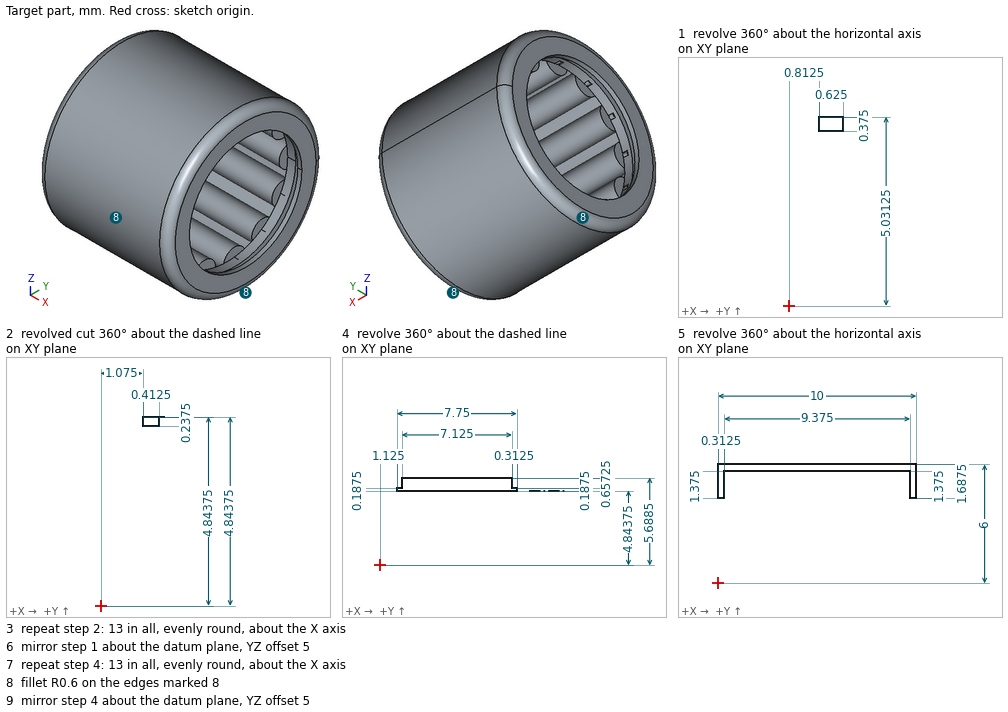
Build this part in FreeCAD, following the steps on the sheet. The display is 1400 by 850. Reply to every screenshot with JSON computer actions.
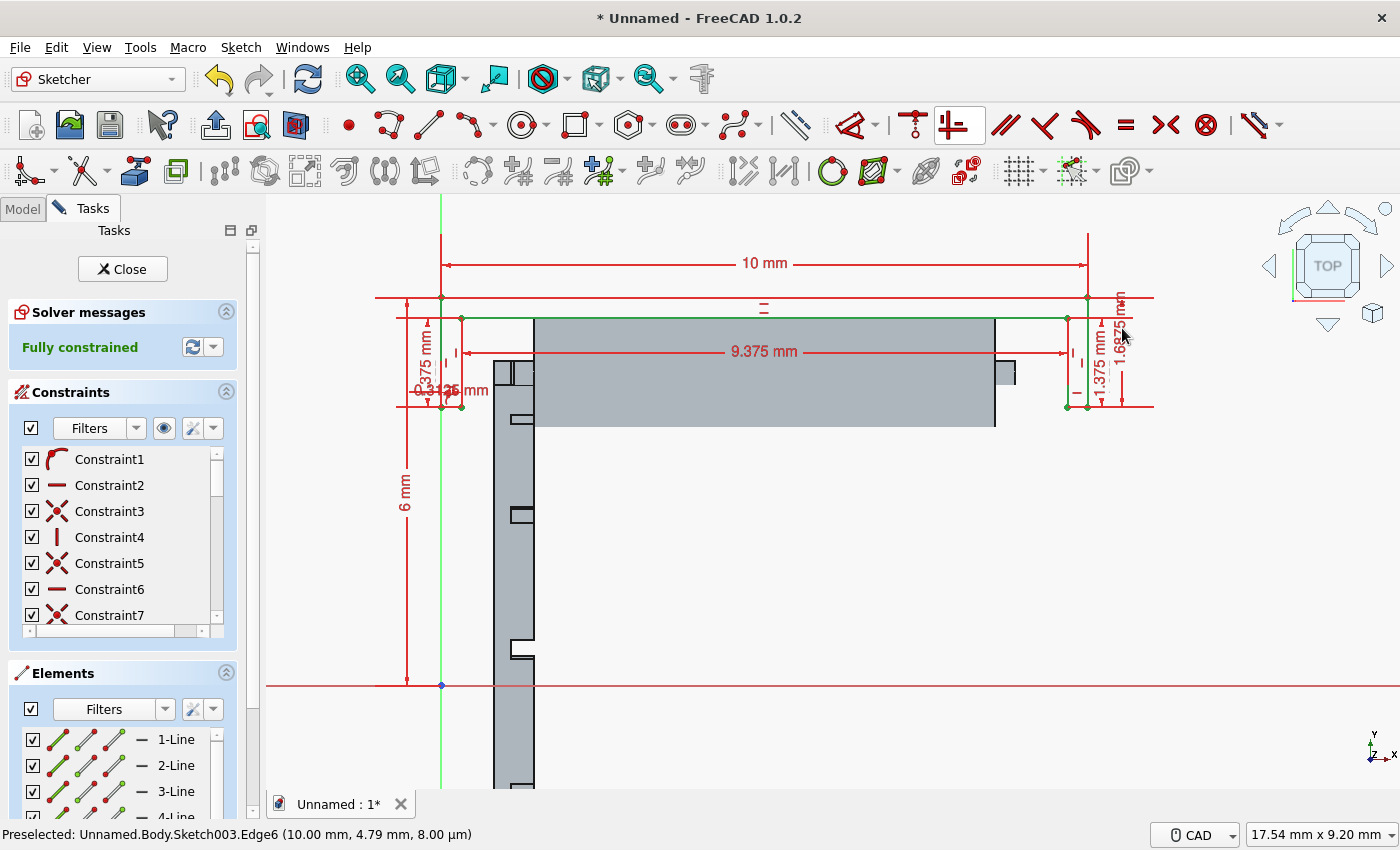
{"action": "left_click", "coordinate": [123, 269]}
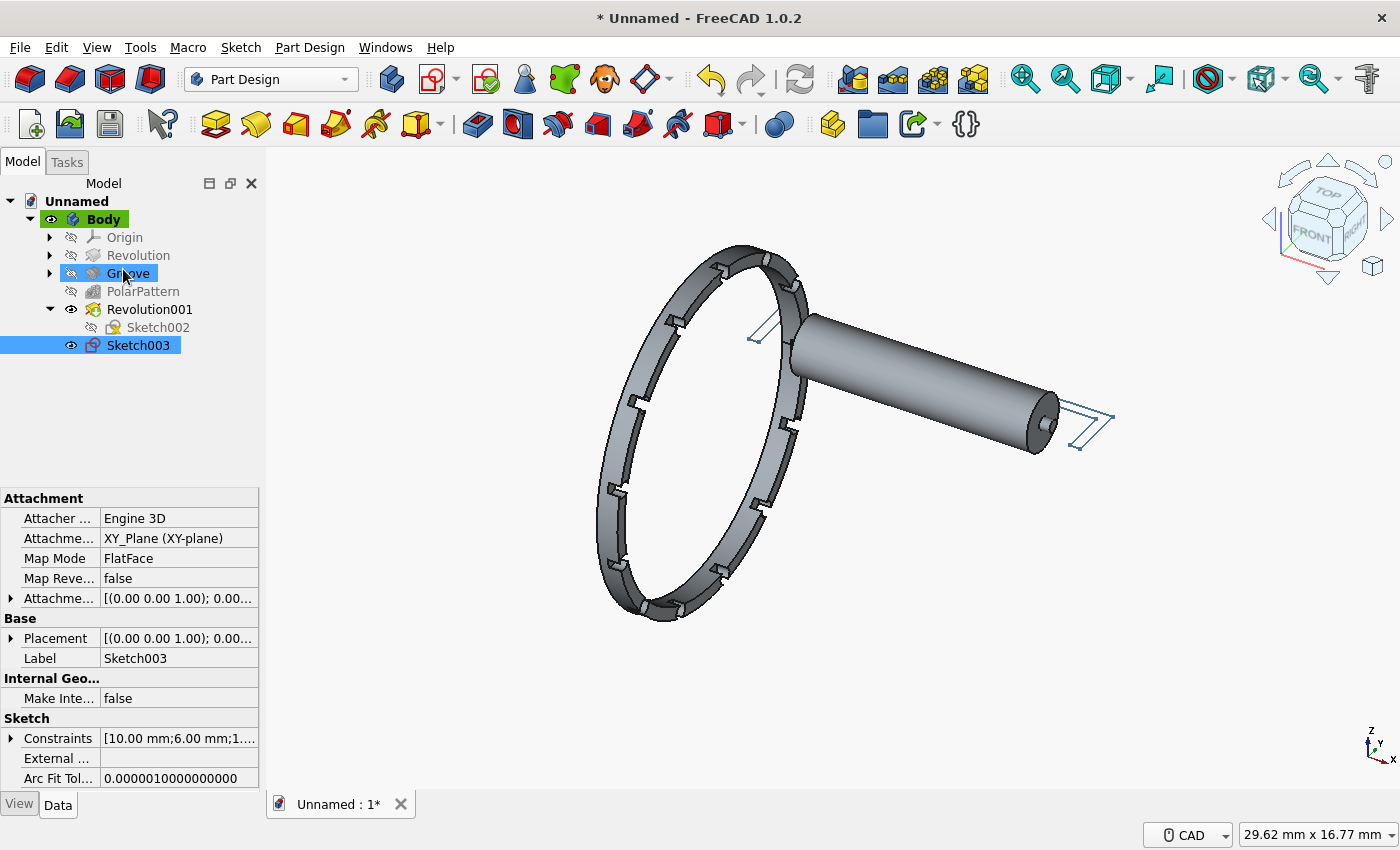
{"action": "left_click", "coordinate": [256, 124]}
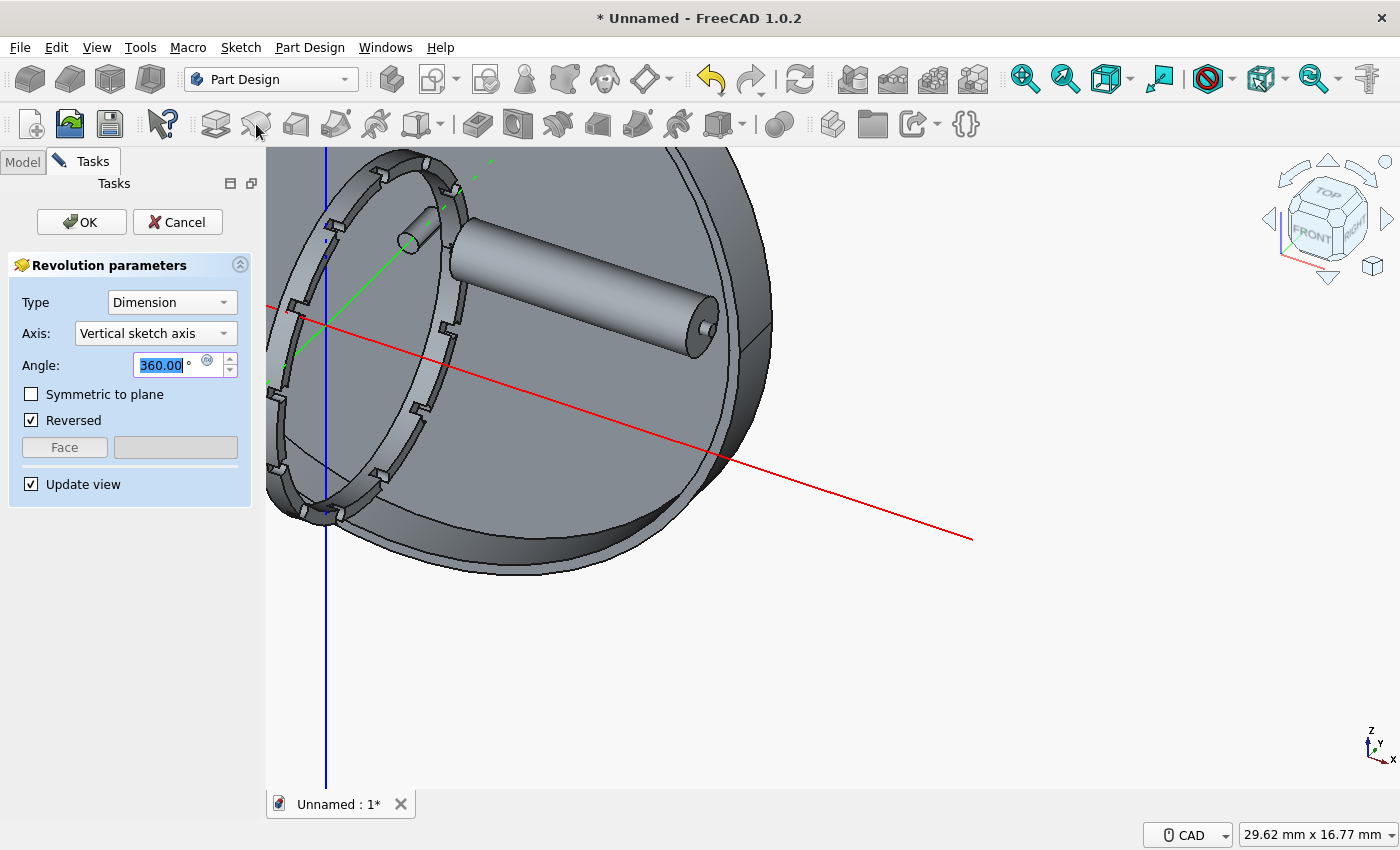
{"action": "left_click", "coordinate": [156, 334]}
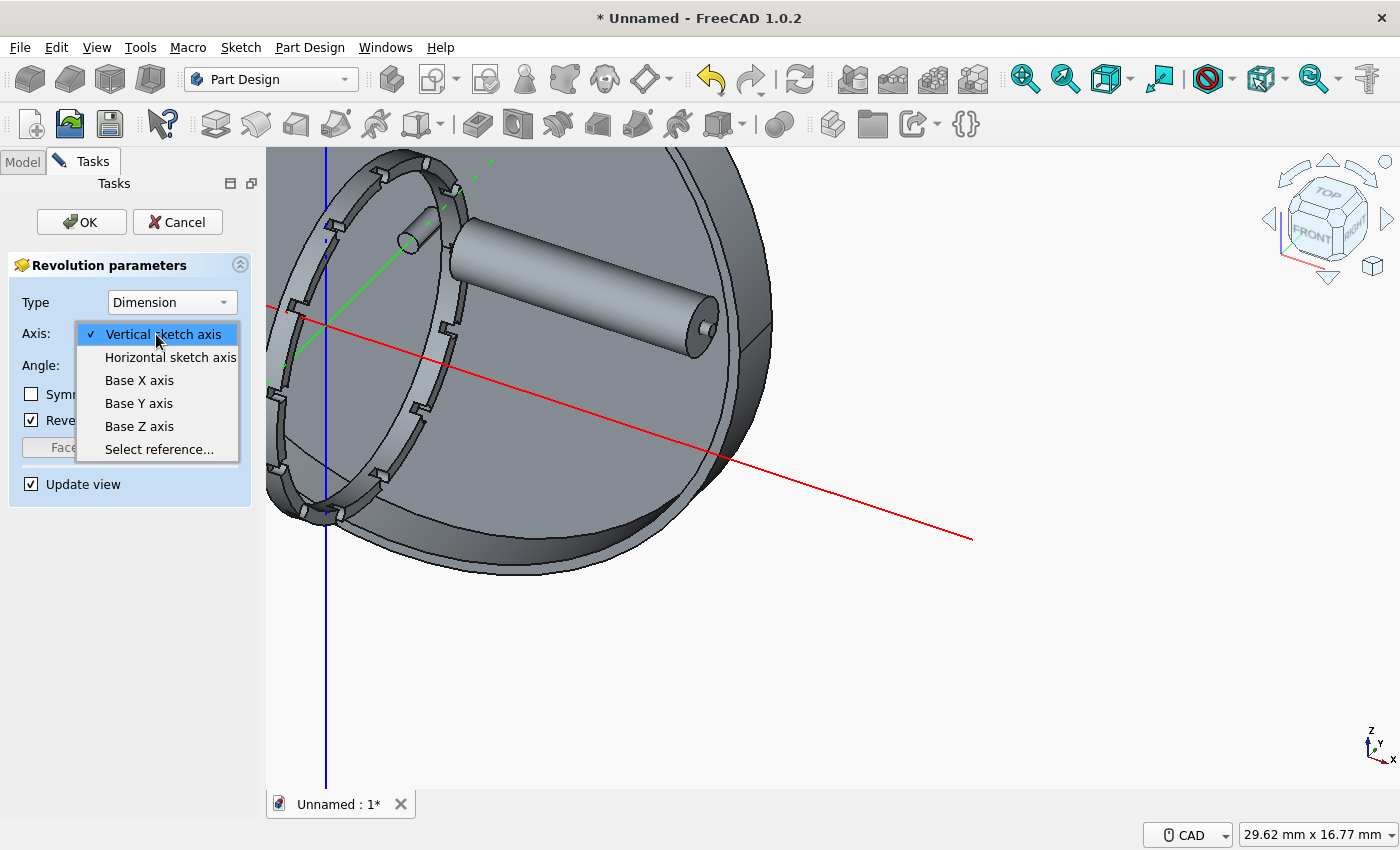
{"action": "left_click", "coordinate": [156, 358]}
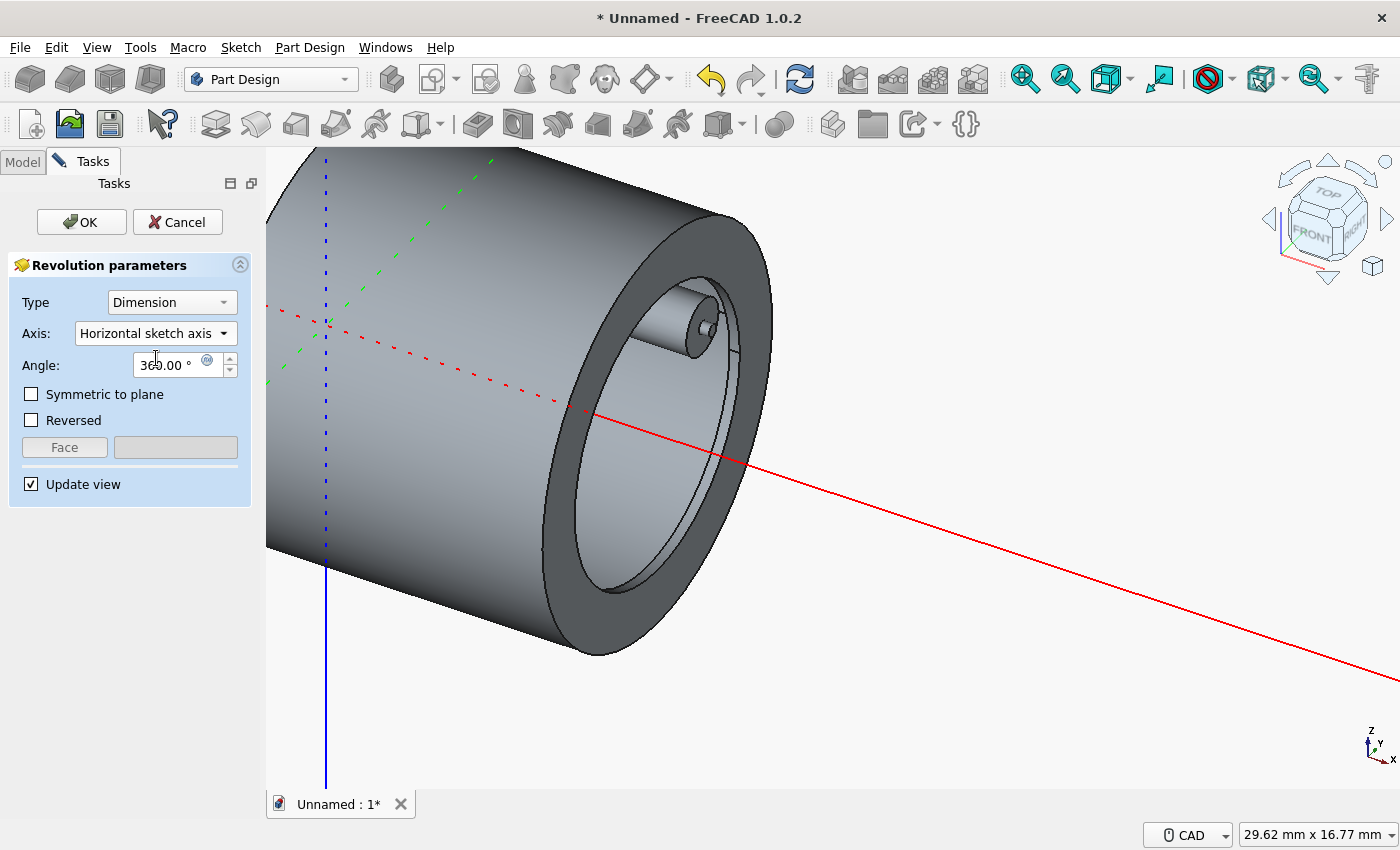
{"action": "left_click", "coordinate": [82, 222]}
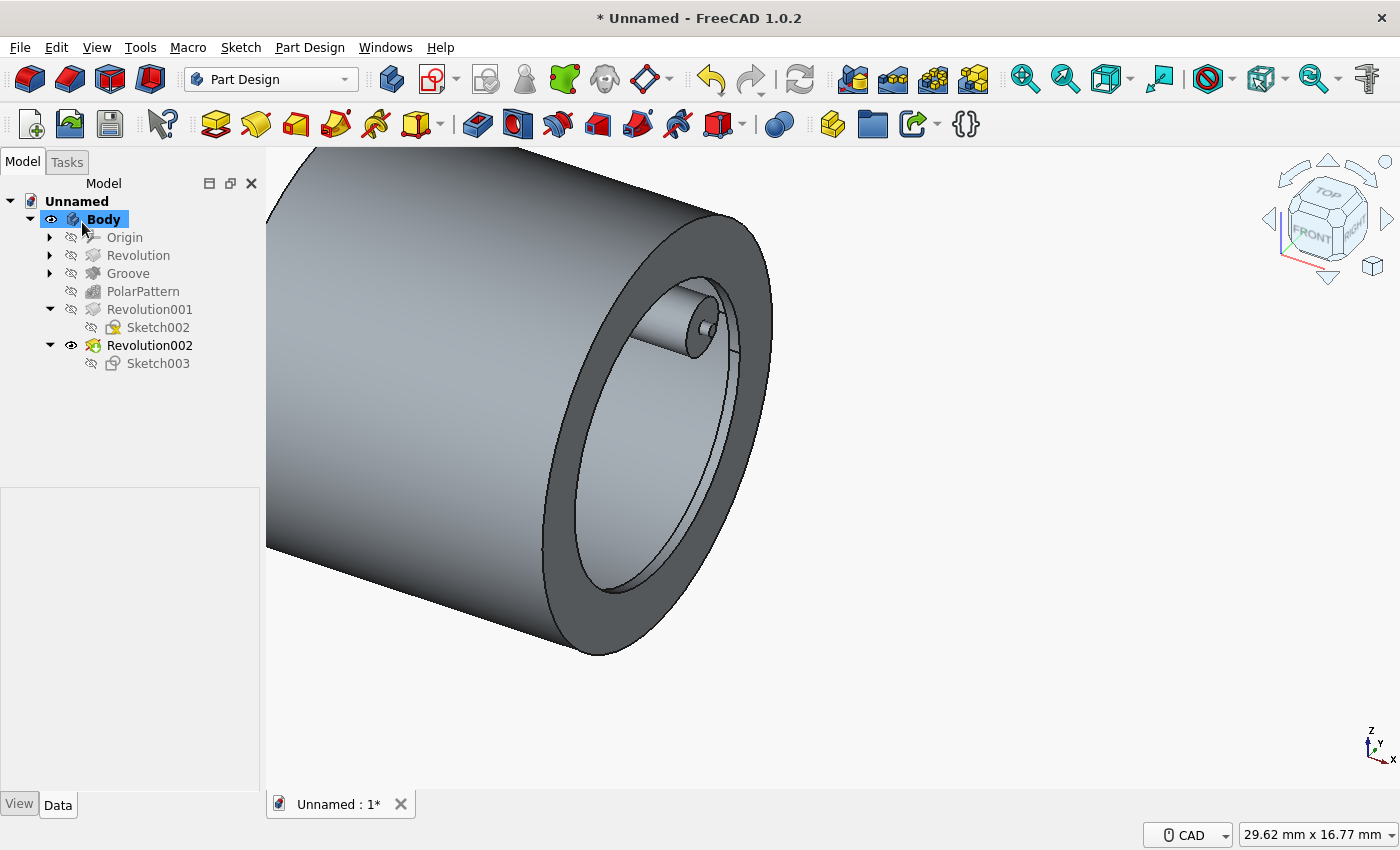
{"action": "key", "text": "v f"}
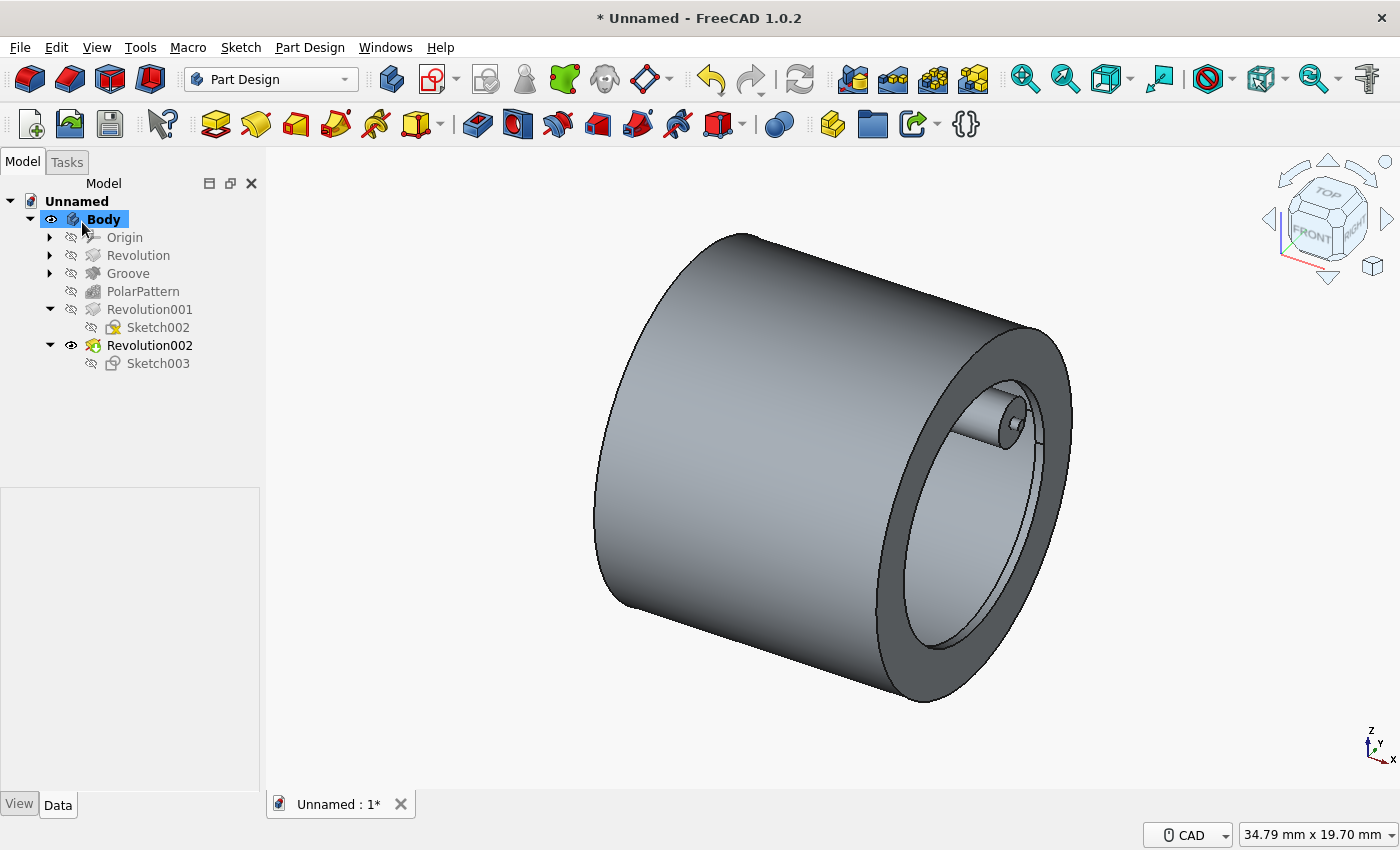
{"action": "left_click", "coordinate": [50, 237]}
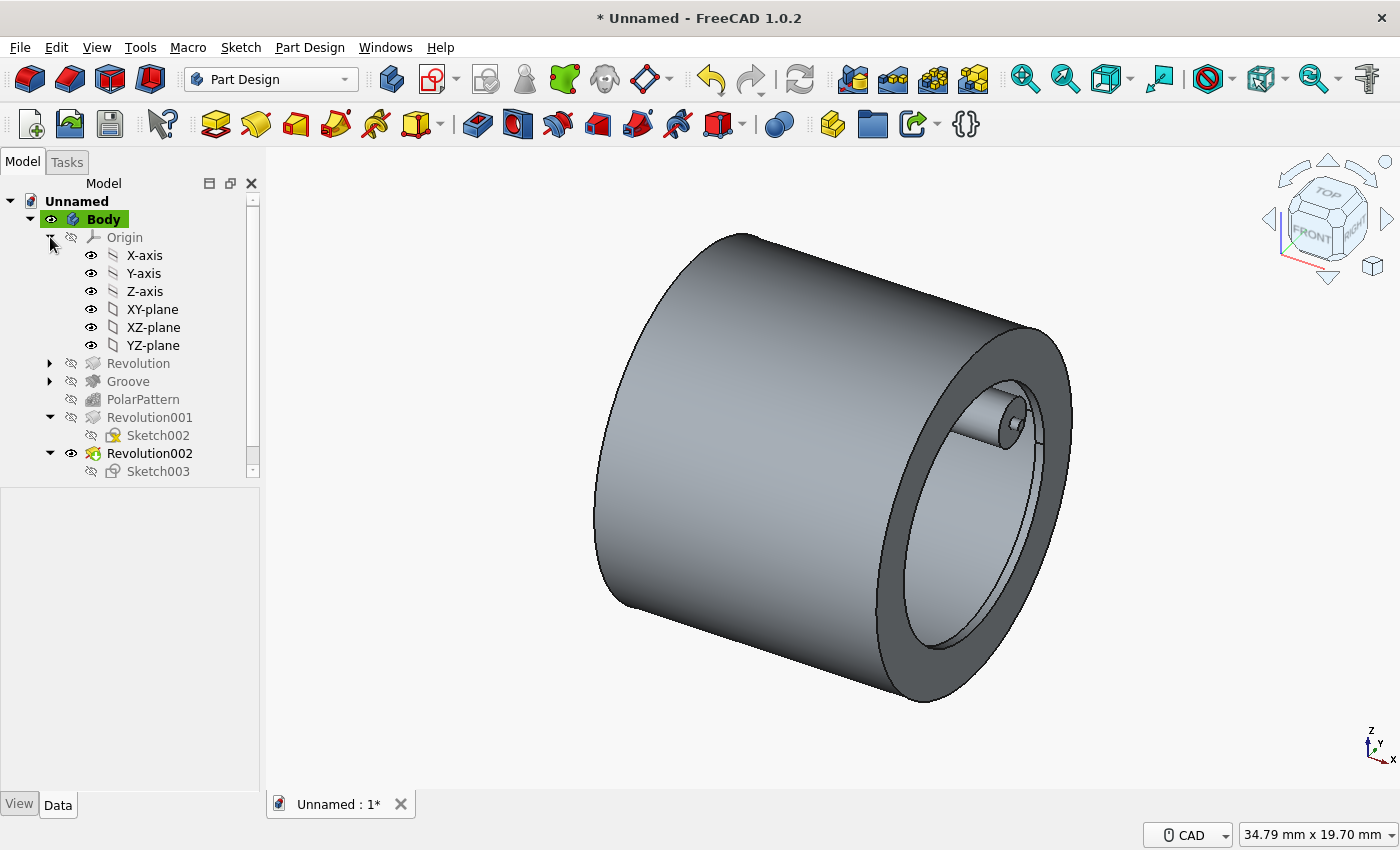
{"action": "left_click", "coordinate": [136, 345]}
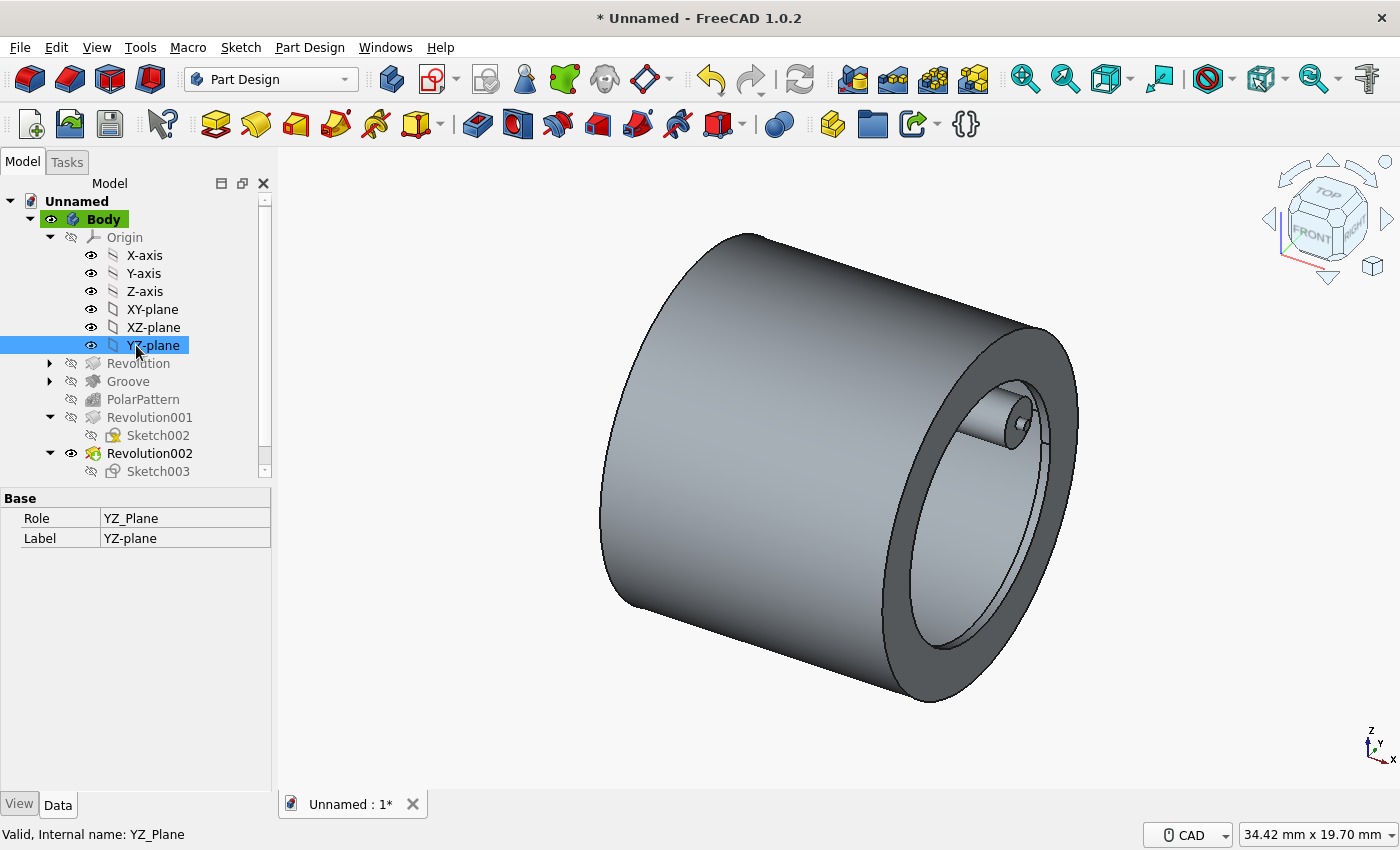
{"action": "left_click", "coordinate": [646, 80]}